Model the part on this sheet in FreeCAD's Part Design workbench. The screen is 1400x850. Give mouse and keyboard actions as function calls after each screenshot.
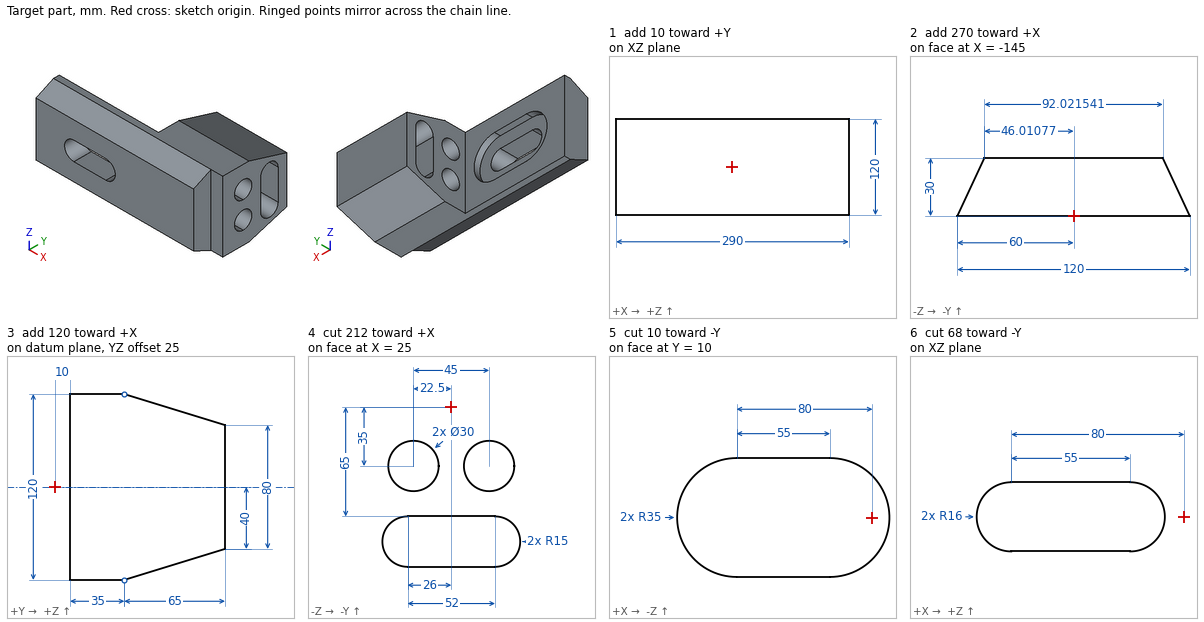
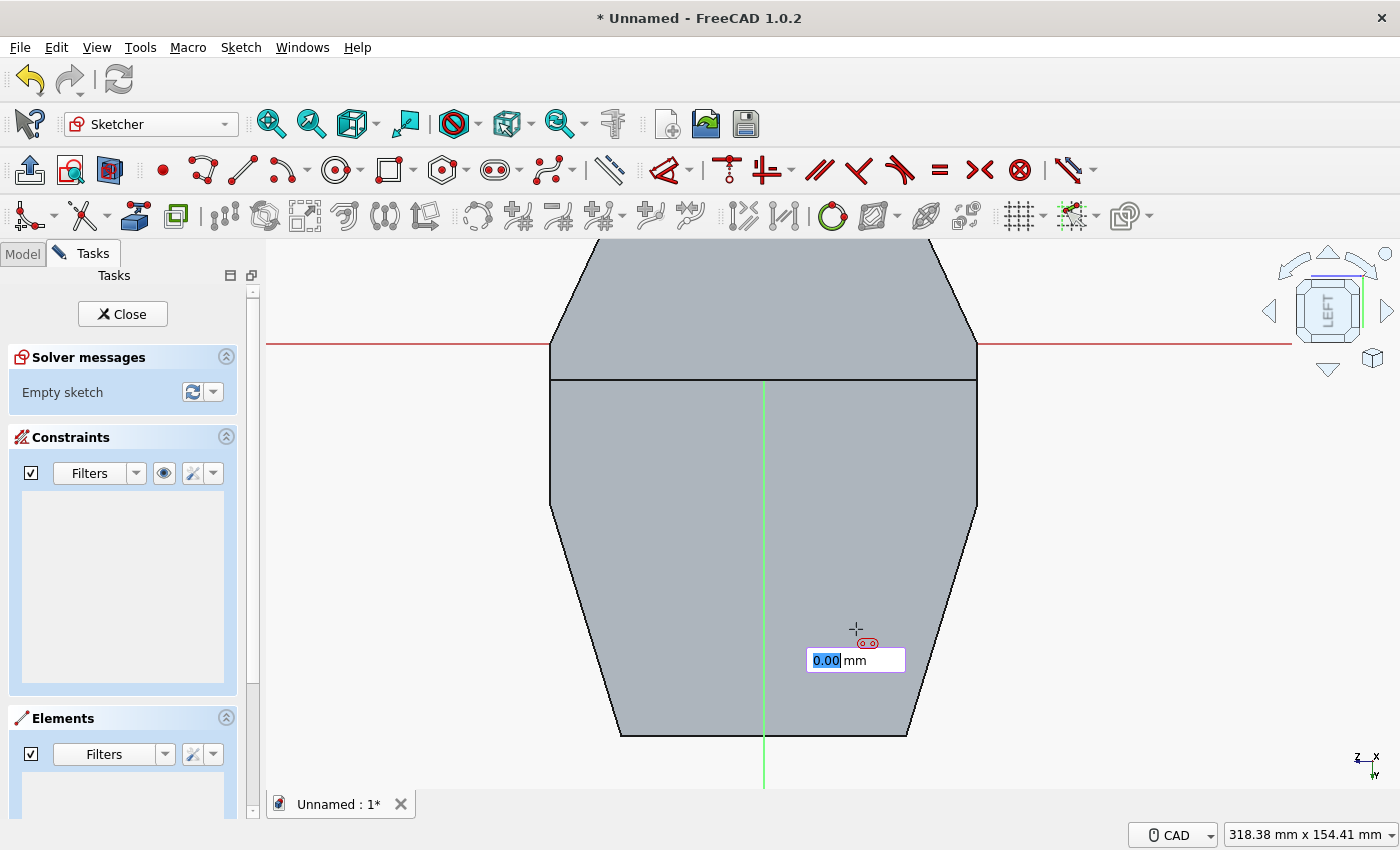
click(736, 682)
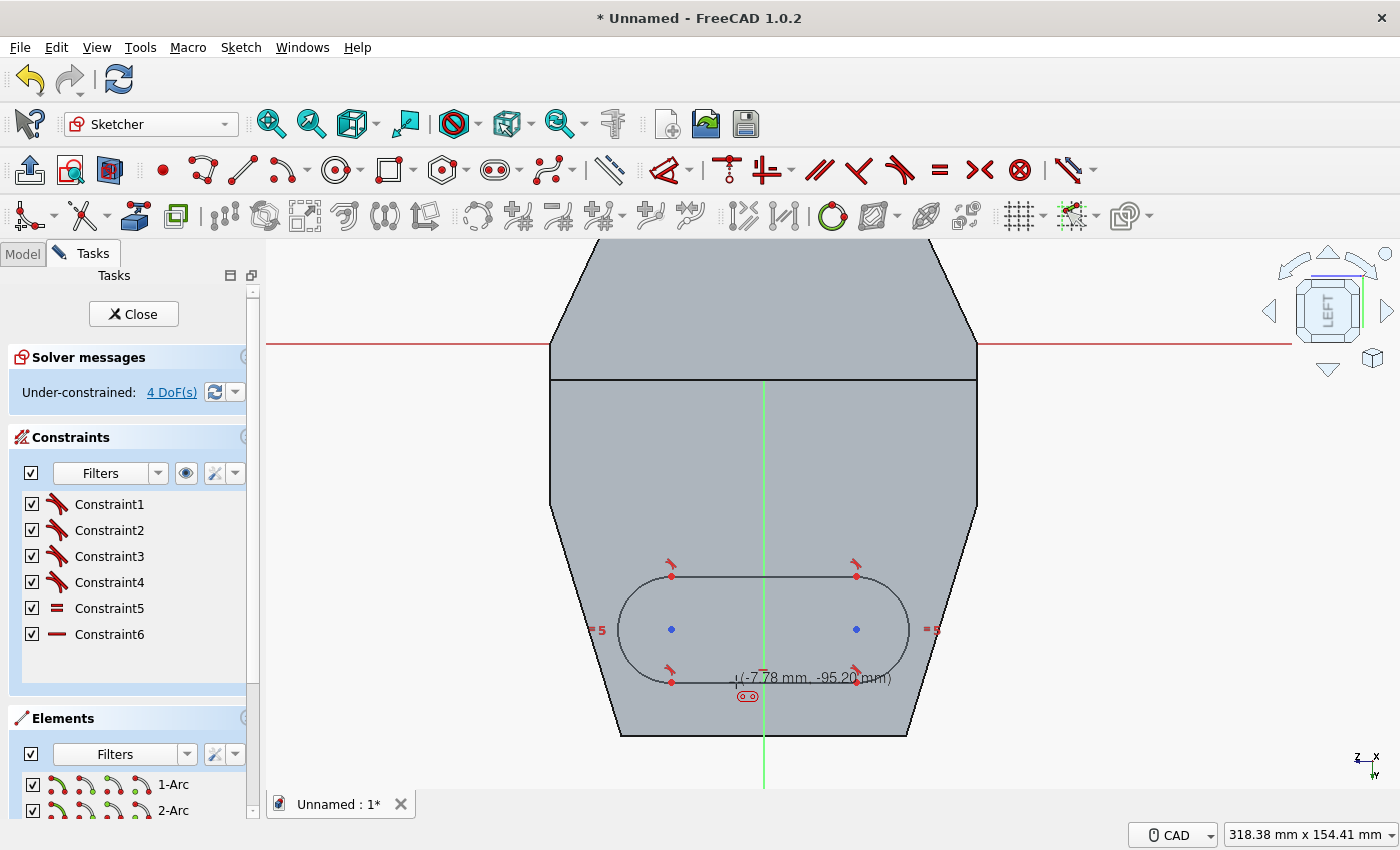
key(g)
key(c)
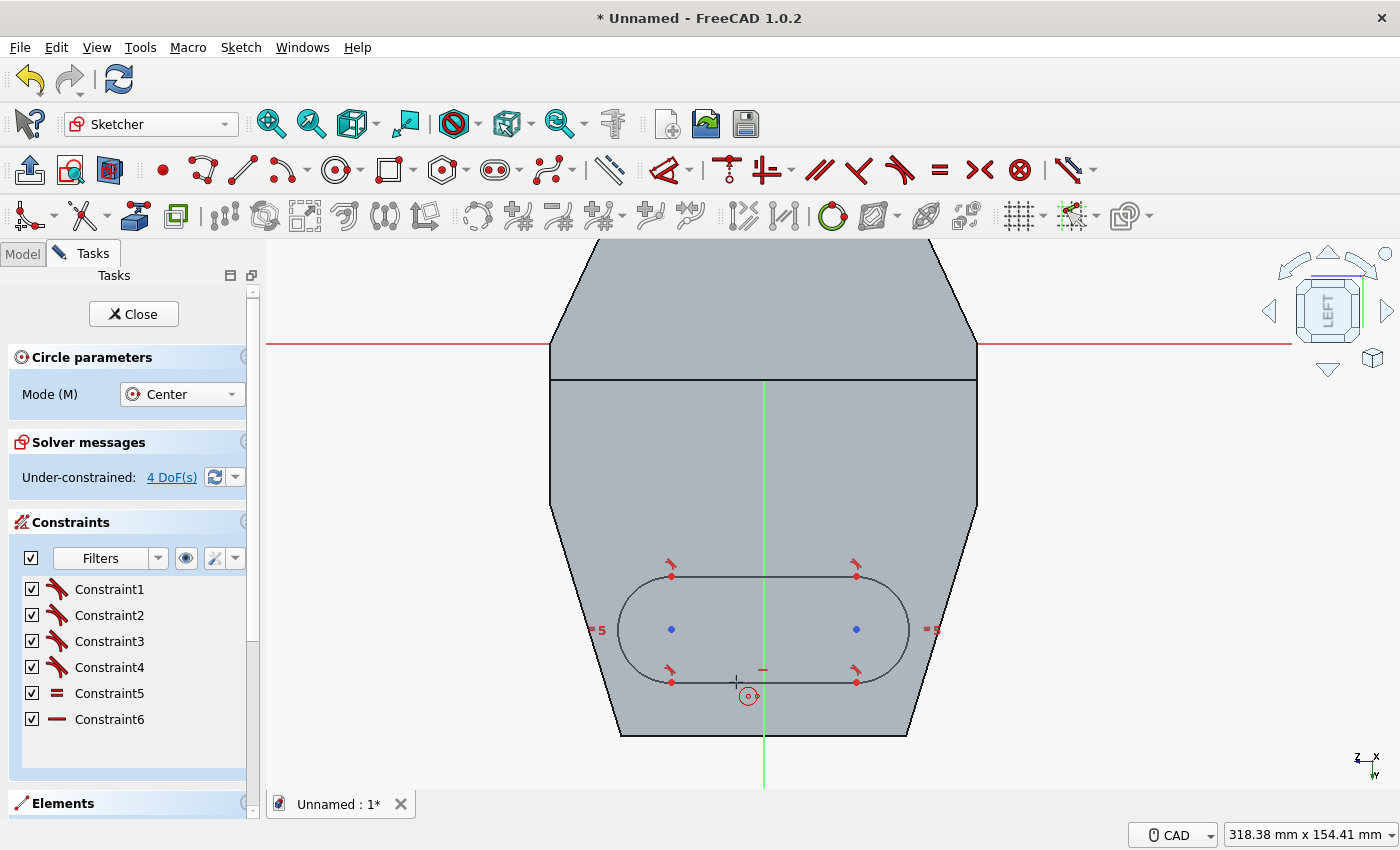
click(684, 469)
click(721, 431)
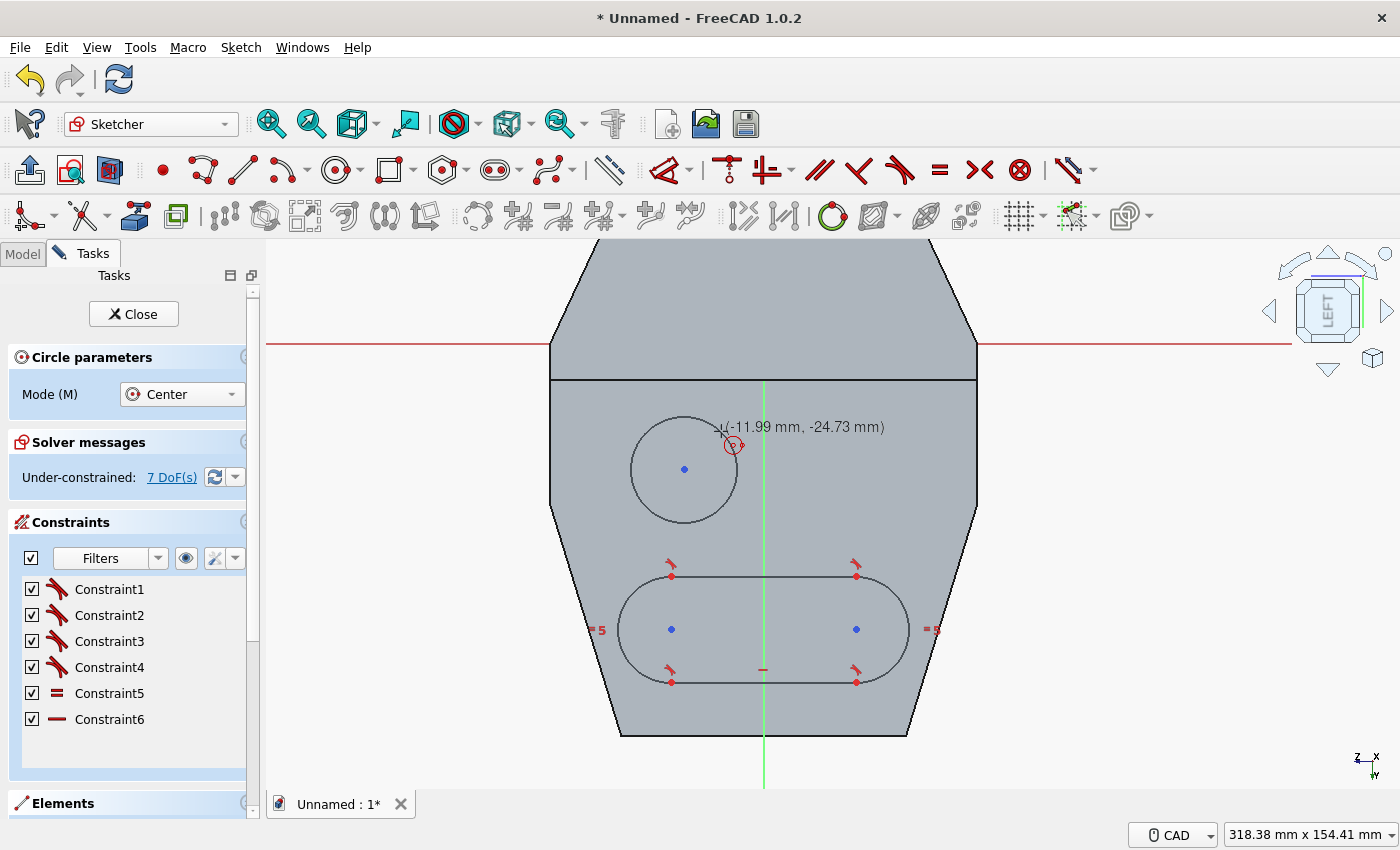
click(844, 469)
click(882, 431)
key(Escape)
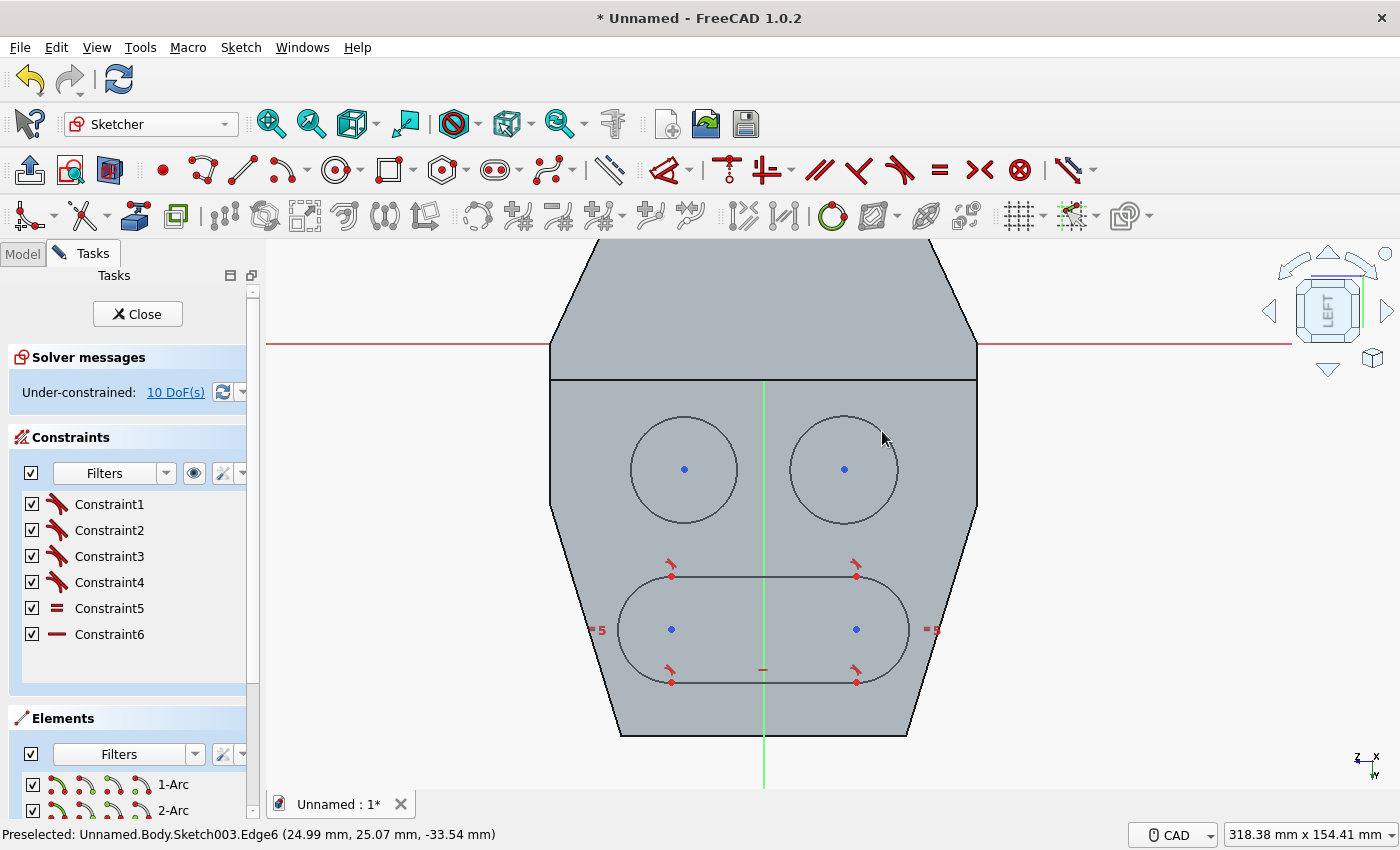
click(721, 432)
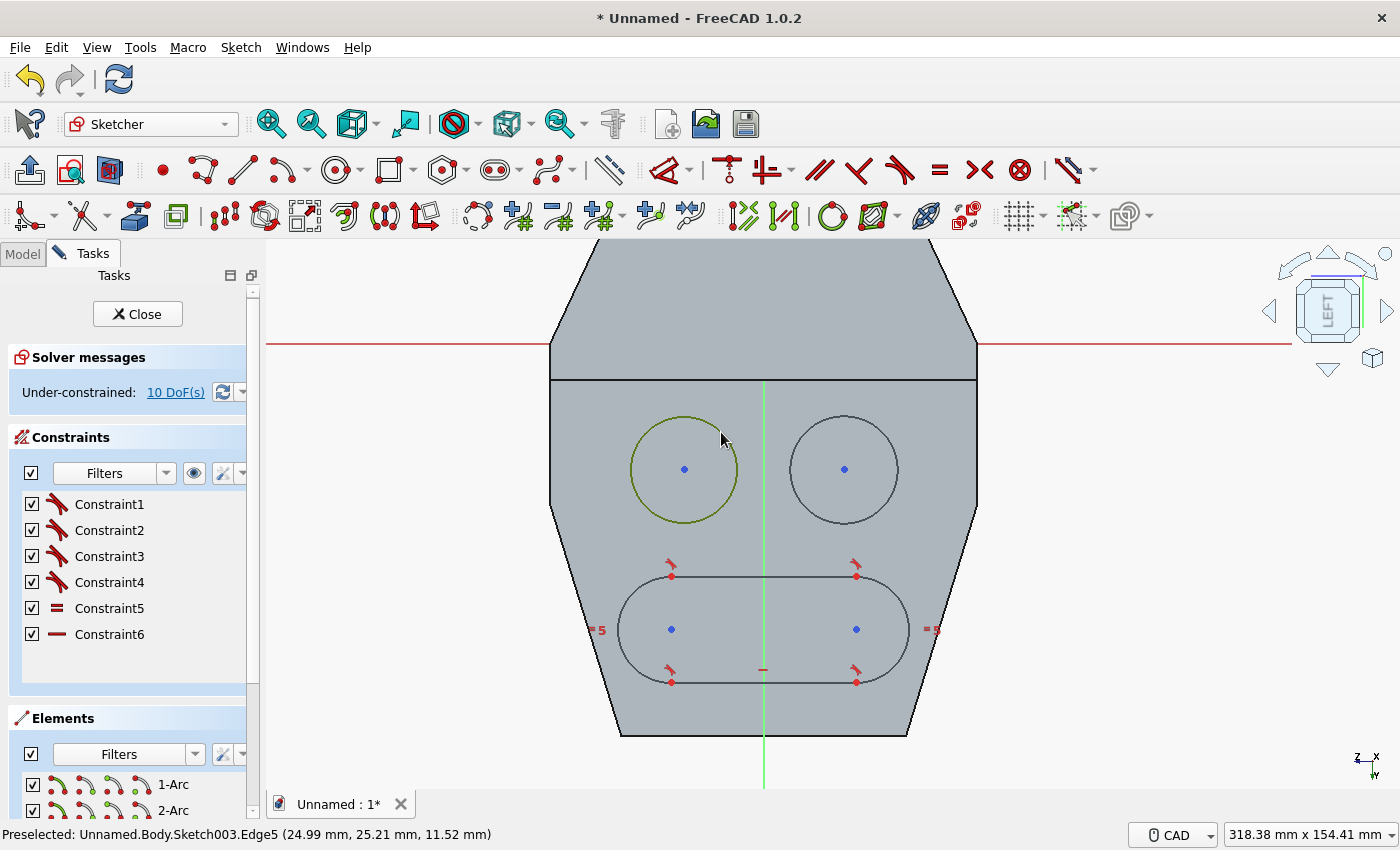
click(882, 432)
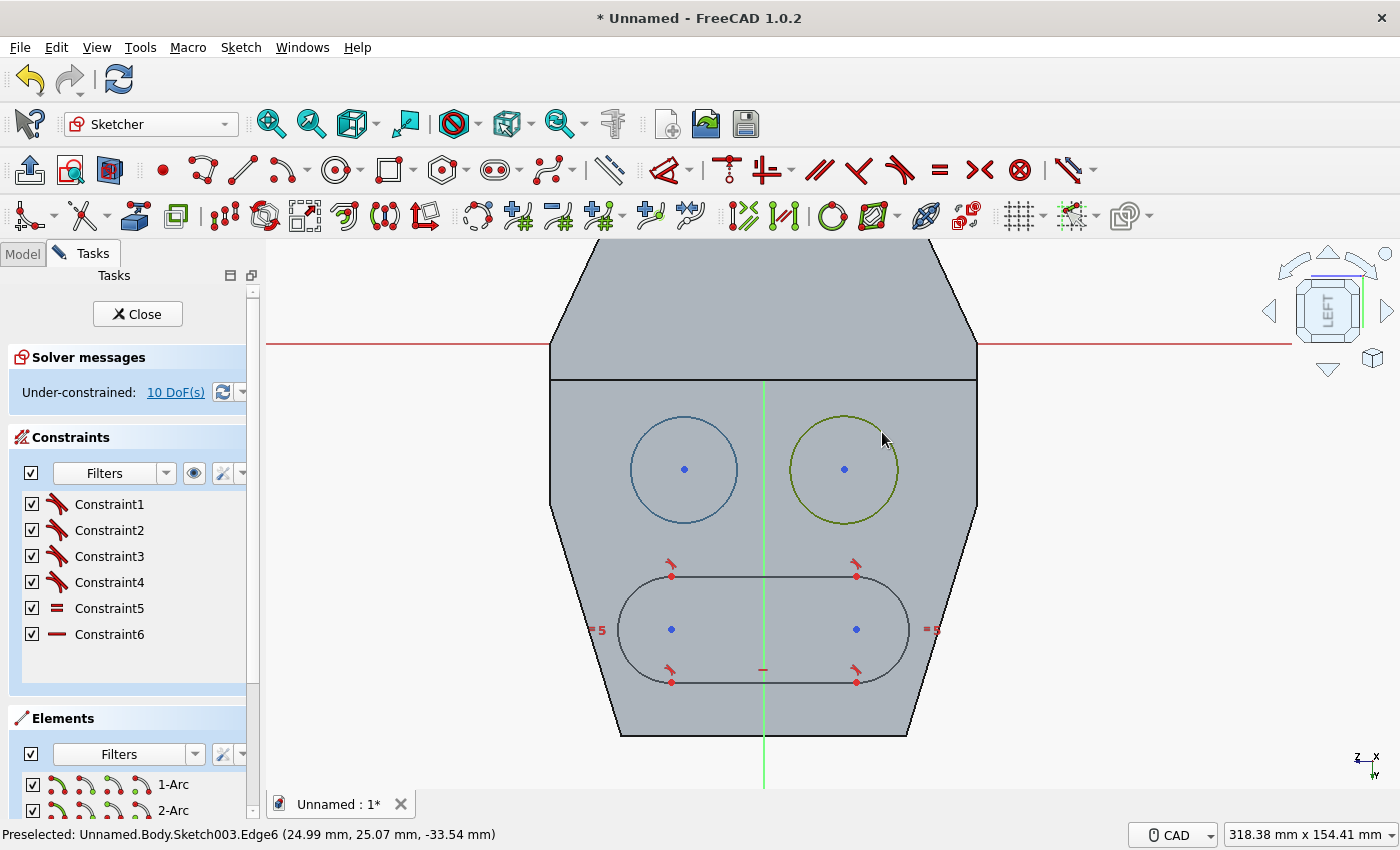
key(e)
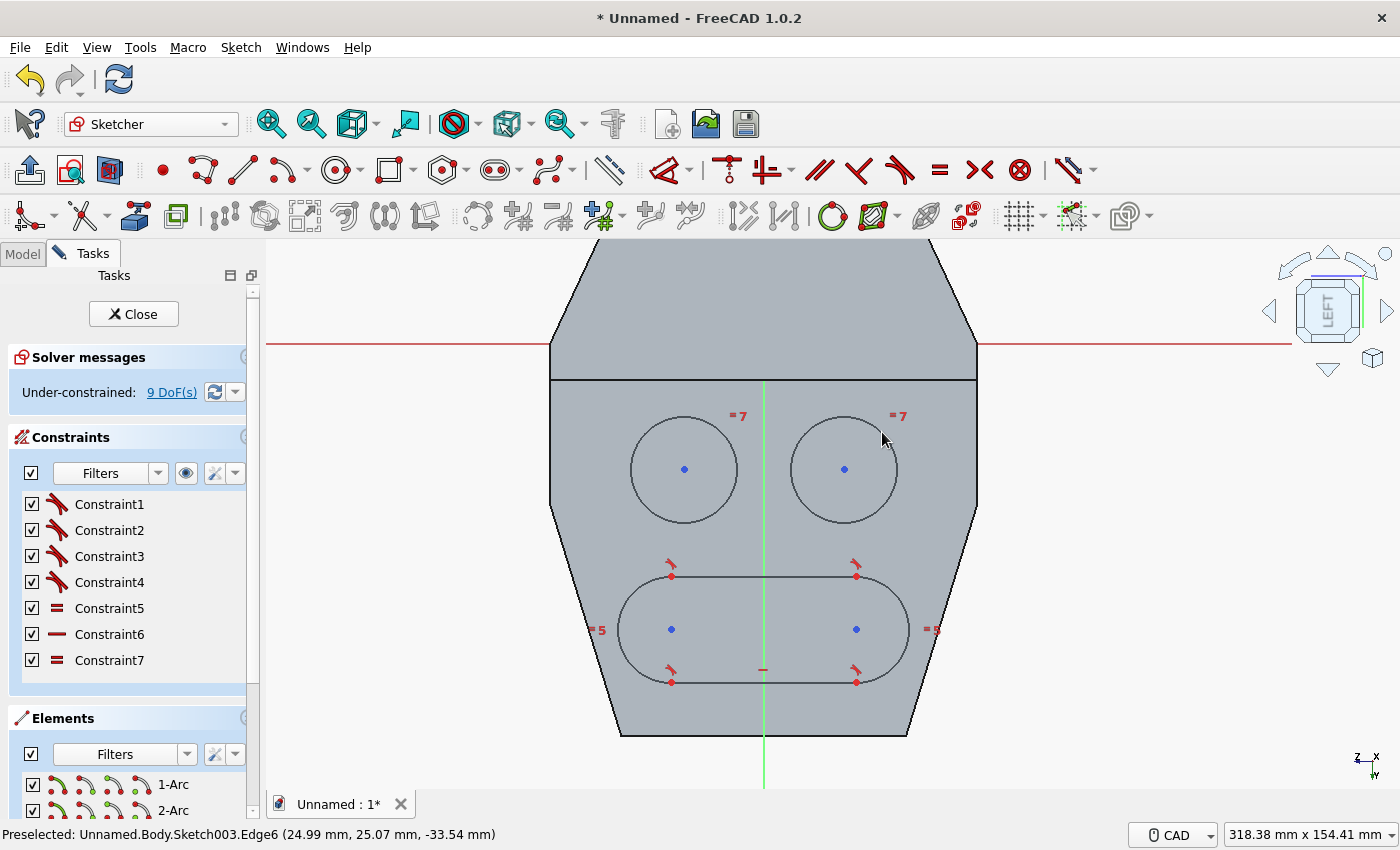
click(684, 470)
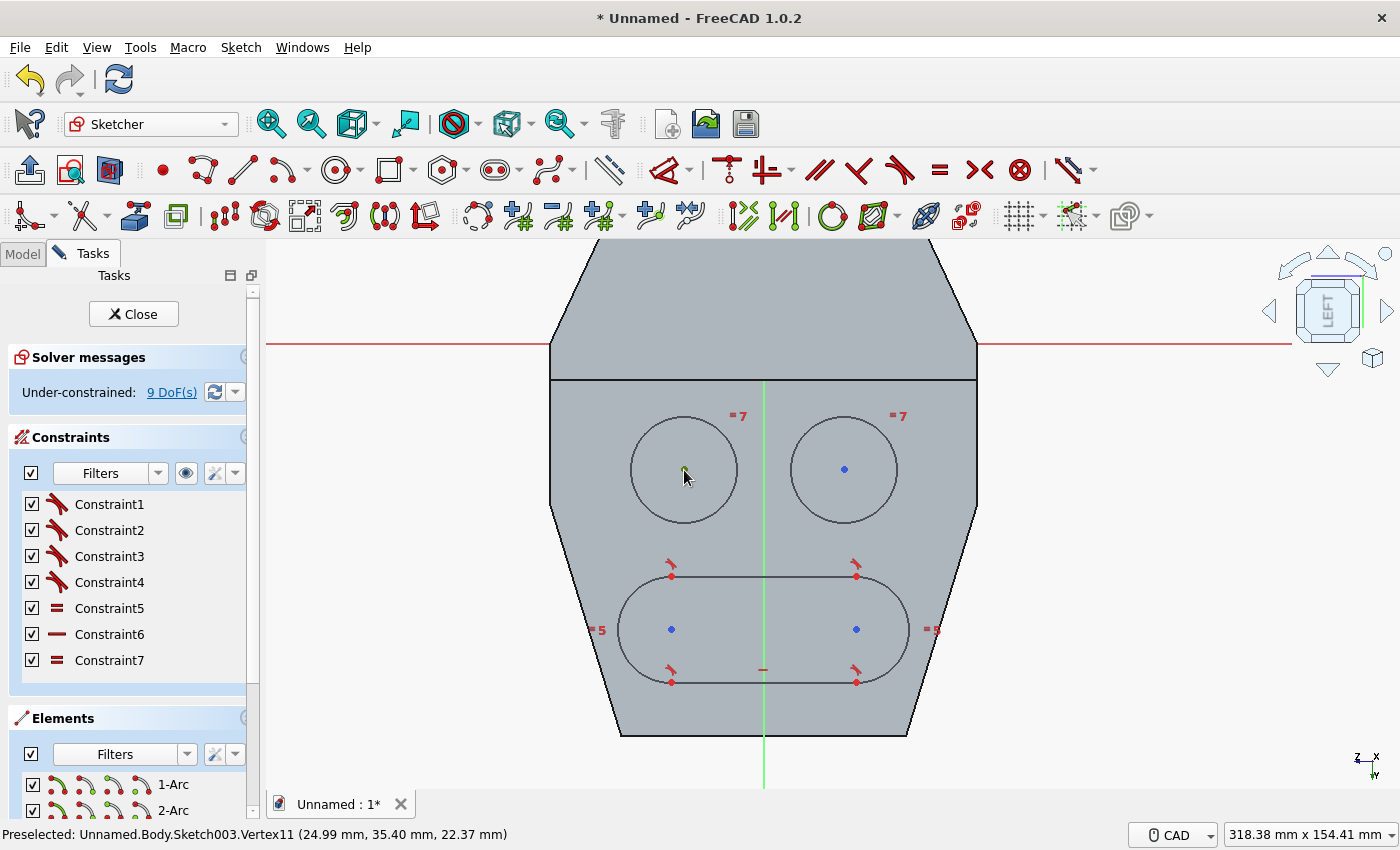
click(844, 470)